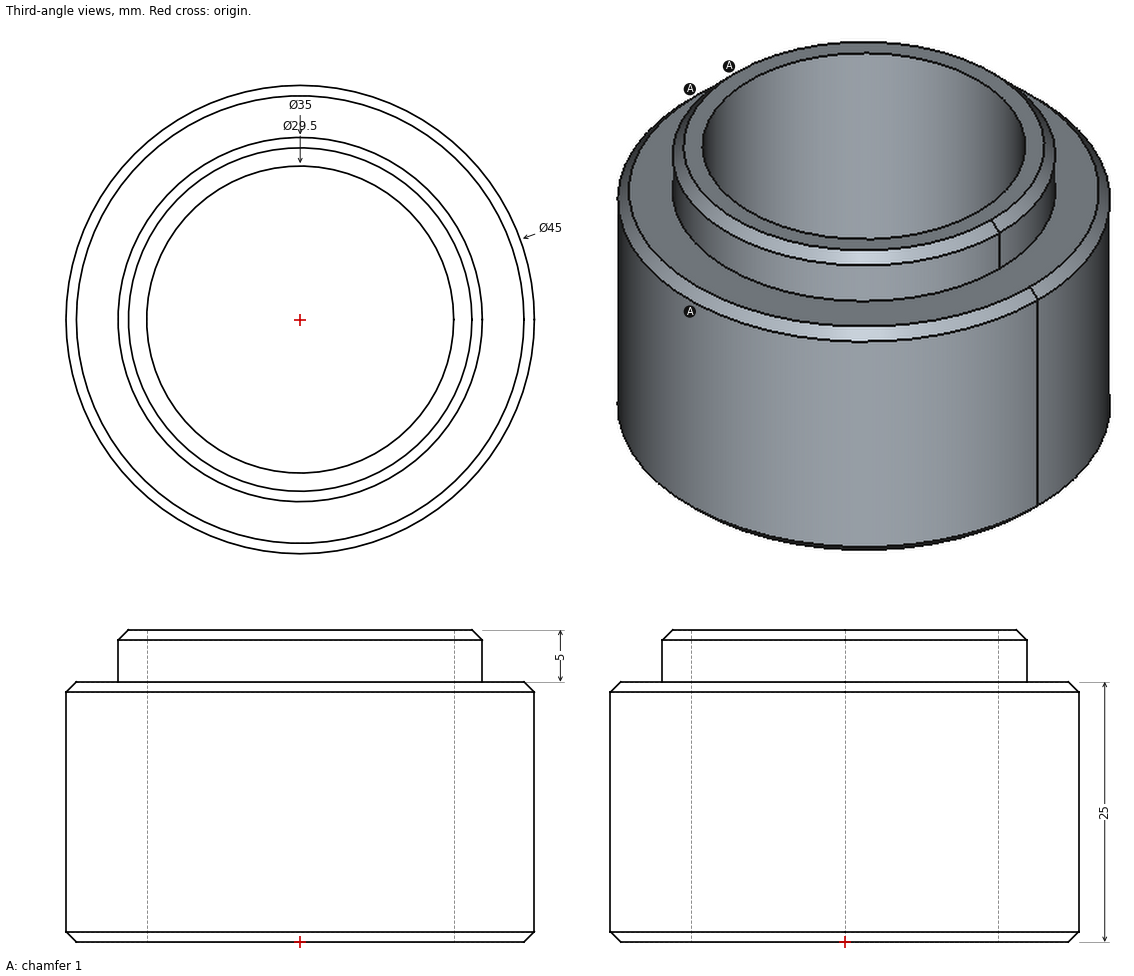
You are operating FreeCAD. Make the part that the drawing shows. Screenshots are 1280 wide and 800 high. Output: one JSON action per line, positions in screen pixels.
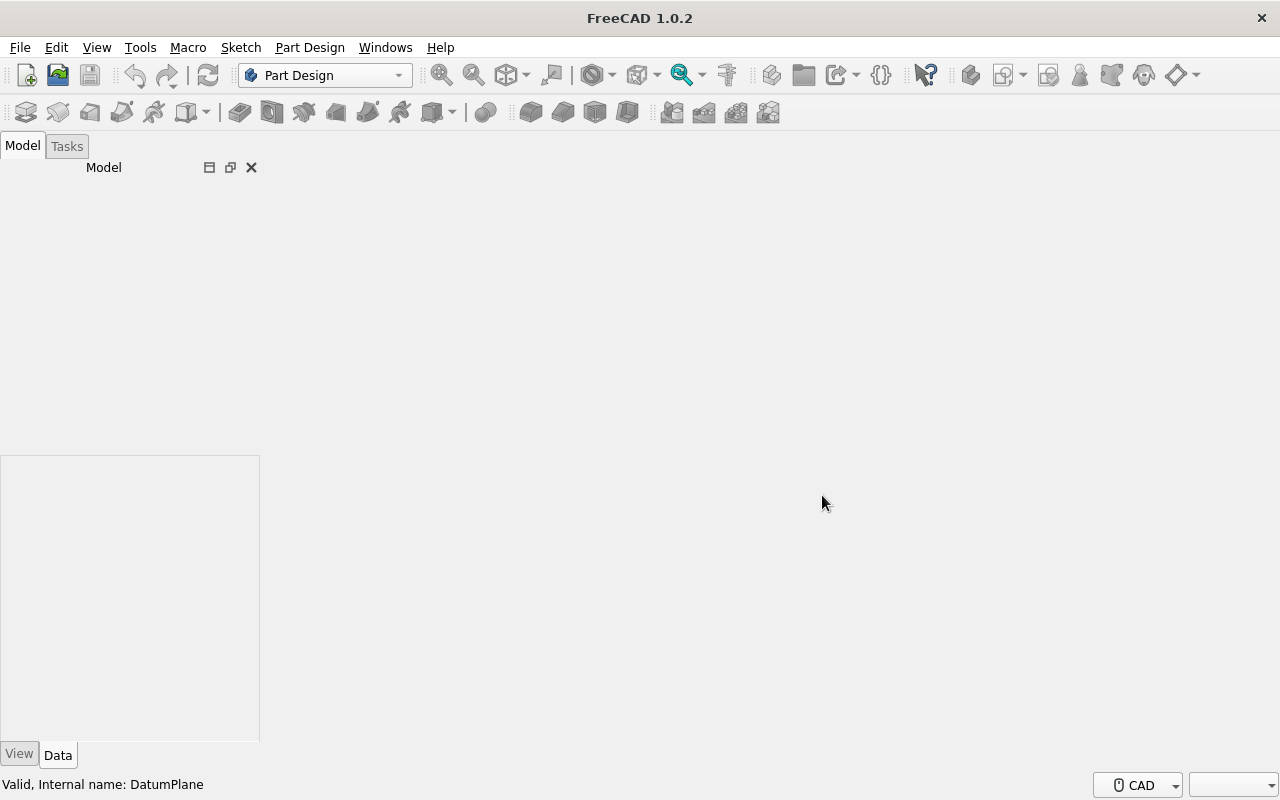
{"action": "left_click", "coordinate": [26, 76]}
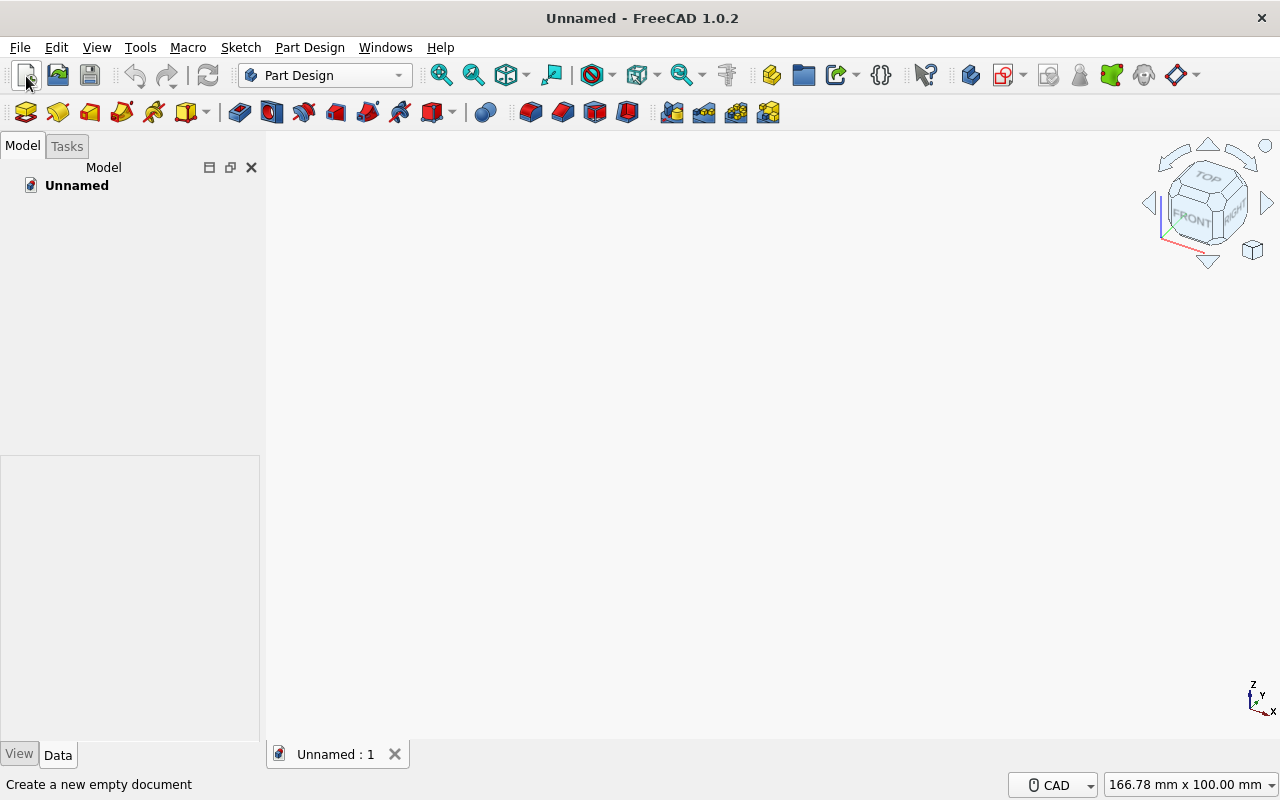
{"action": "left_click", "coordinate": [1004, 76]}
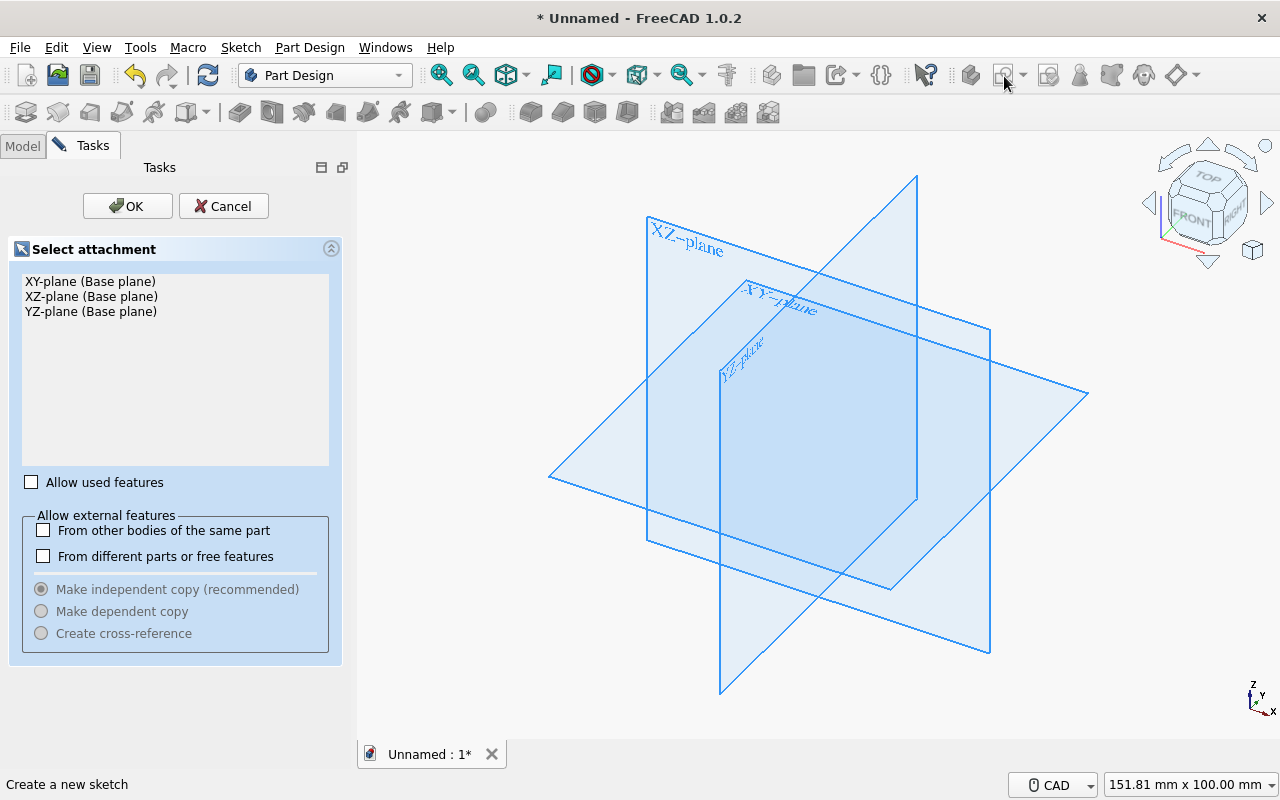
{"action": "left_click", "coordinate": [82, 282]}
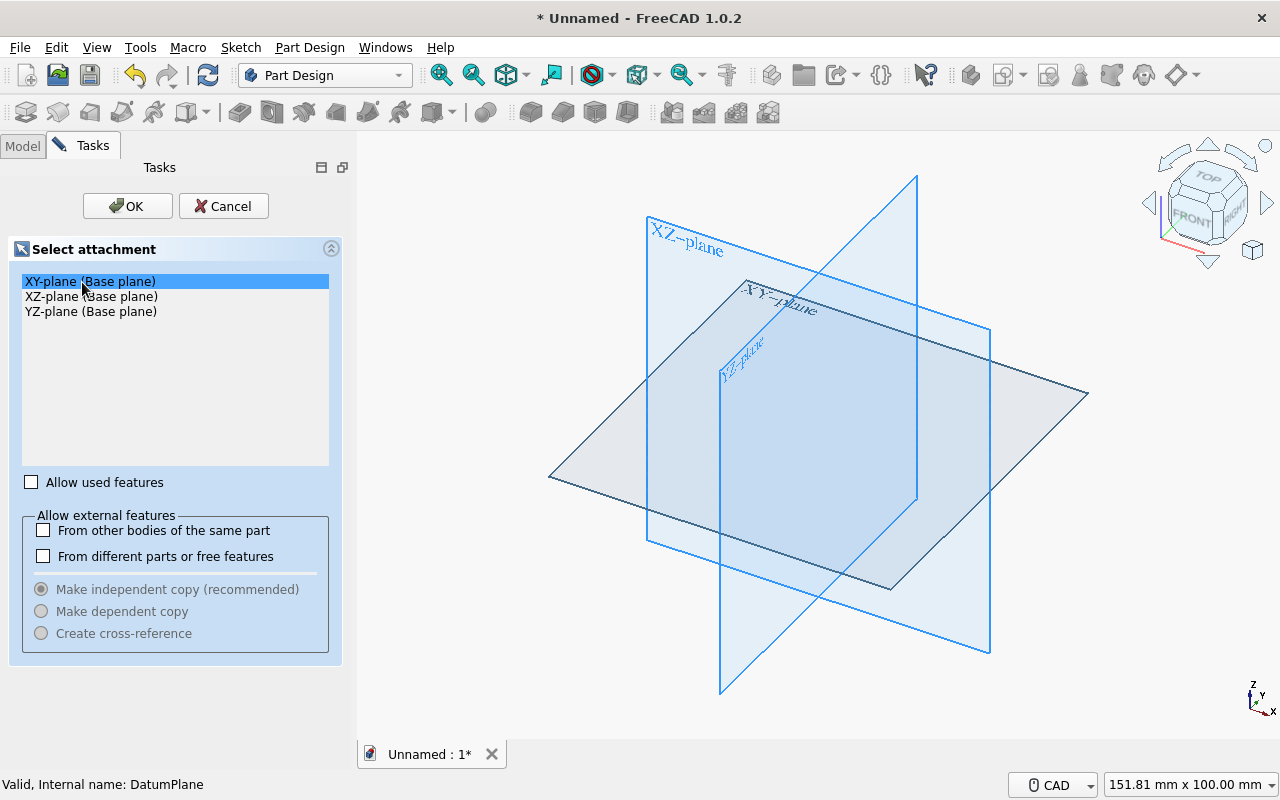
{"action": "left_click", "coordinate": [128, 206]}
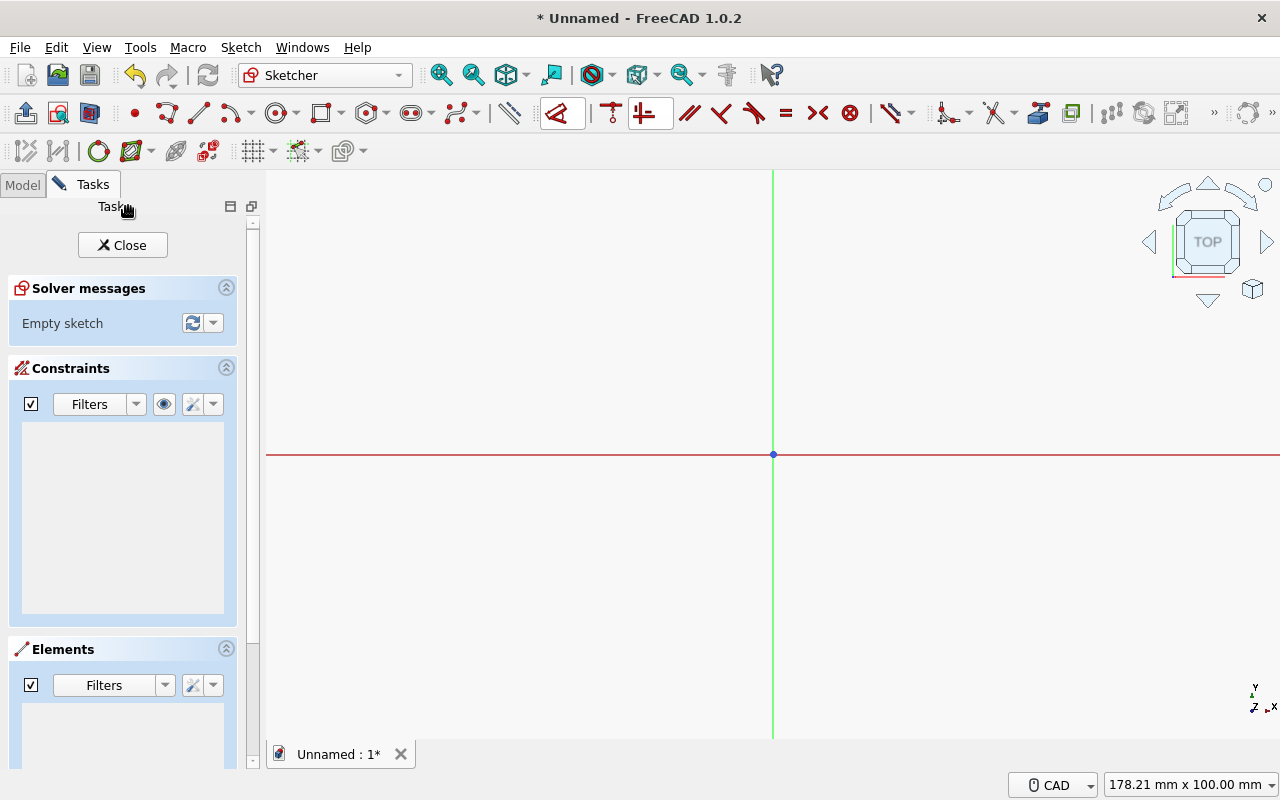
{"action": "scroll", "coordinate": [912, 455], "scroll_direction": "up", "scroll_amount": 2}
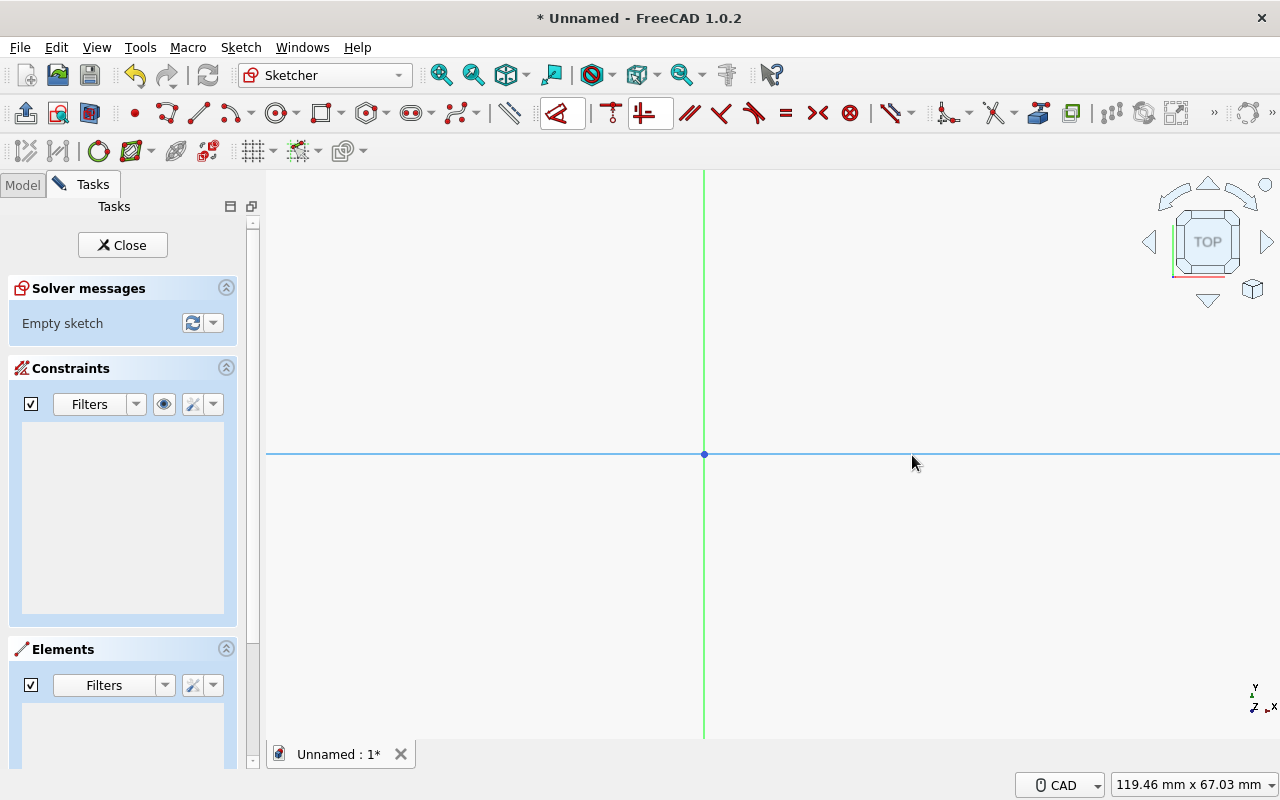
{"action": "left_click", "coordinate": [276, 114]}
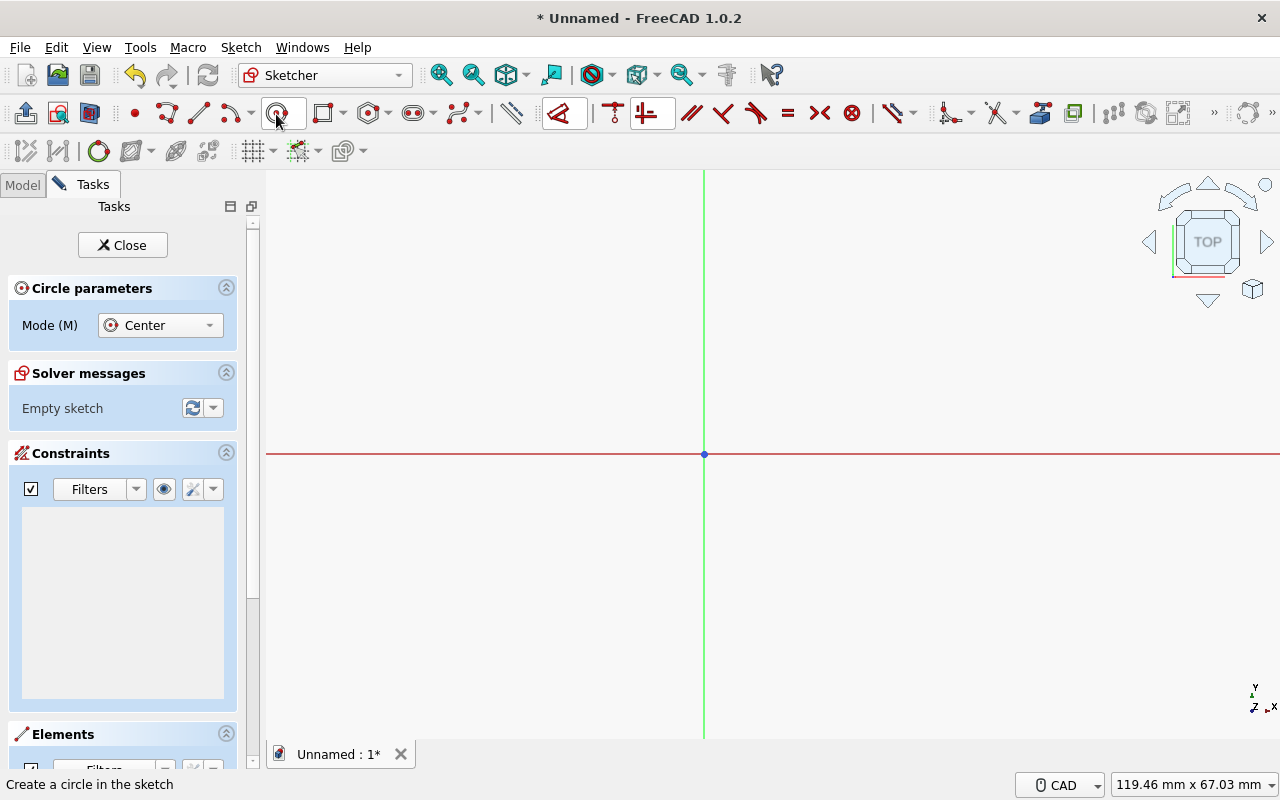
{"action": "left_click", "coordinate": [704, 454]}
{"action": "left_click", "coordinate": [839, 319]}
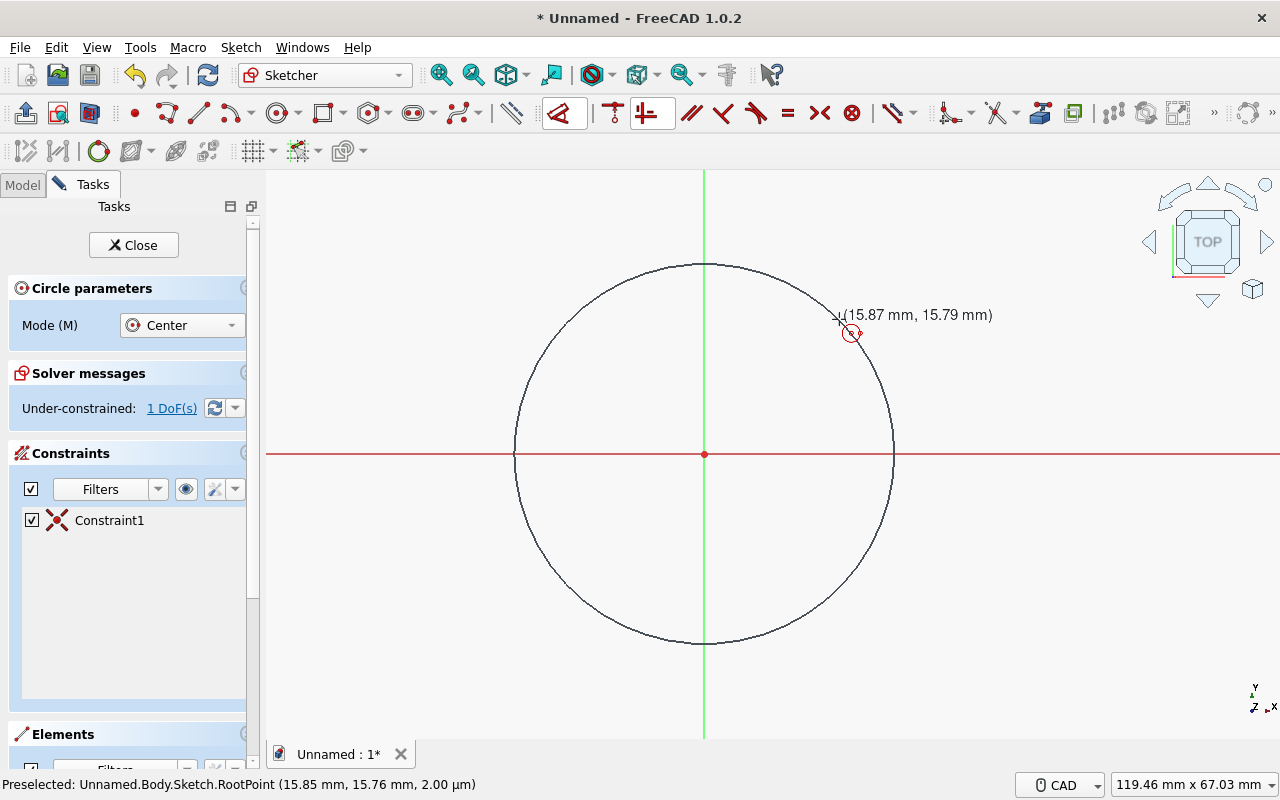
{"action": "left_click", "coordinate": [704, 454]}
{"action": "left_click", "coordinate": [793, 365]}
{"action": "key", "text": "Escape"}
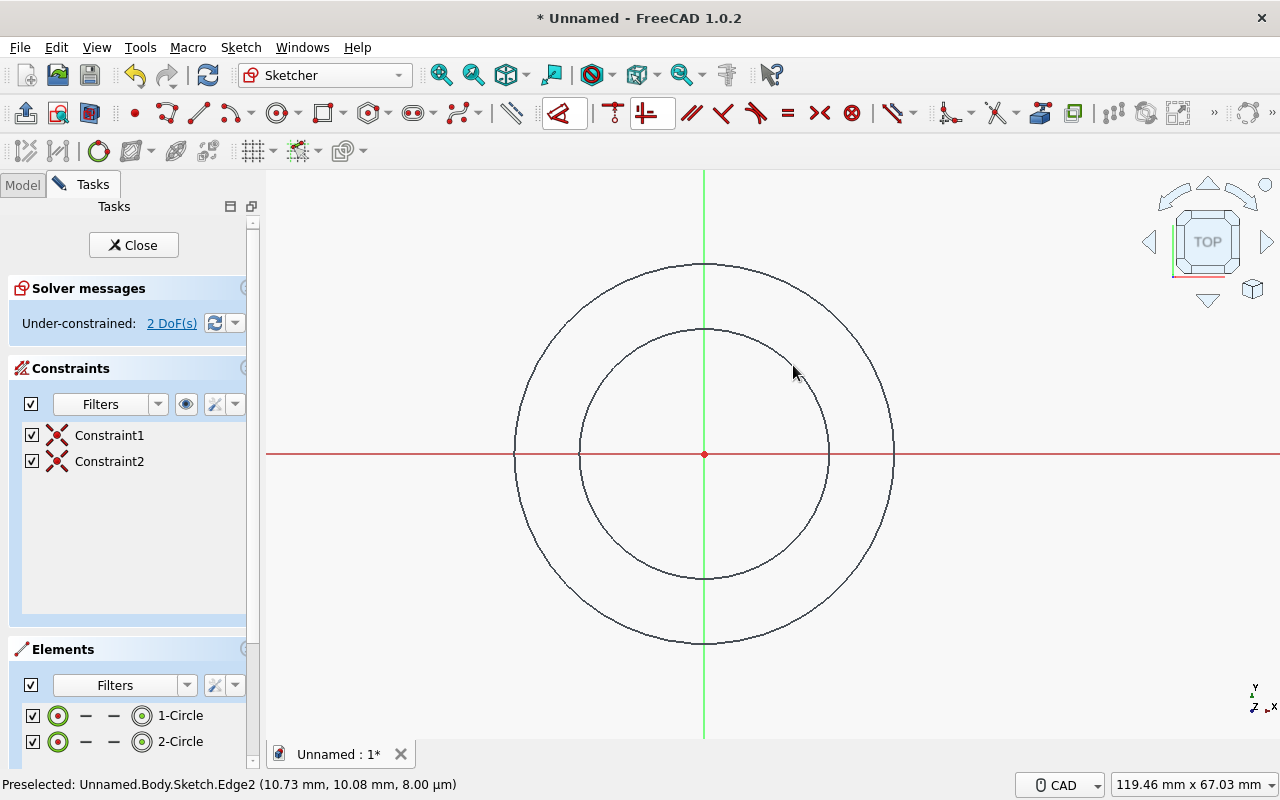
{"action": "left_click", "coordinate": [558, 114]}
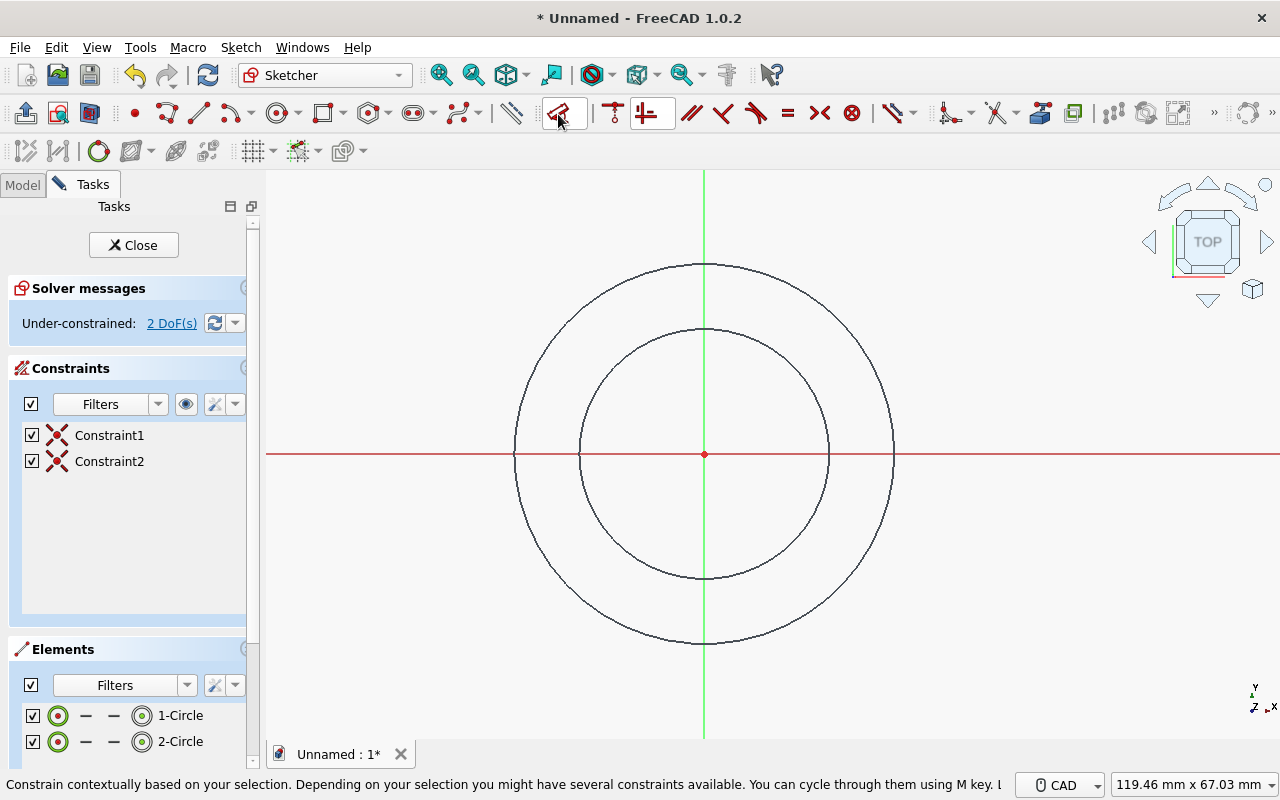
{"action": "left_click", "coordinate": [838, 319]}
{"action": "left_click", "coordinate": [861, 296]}